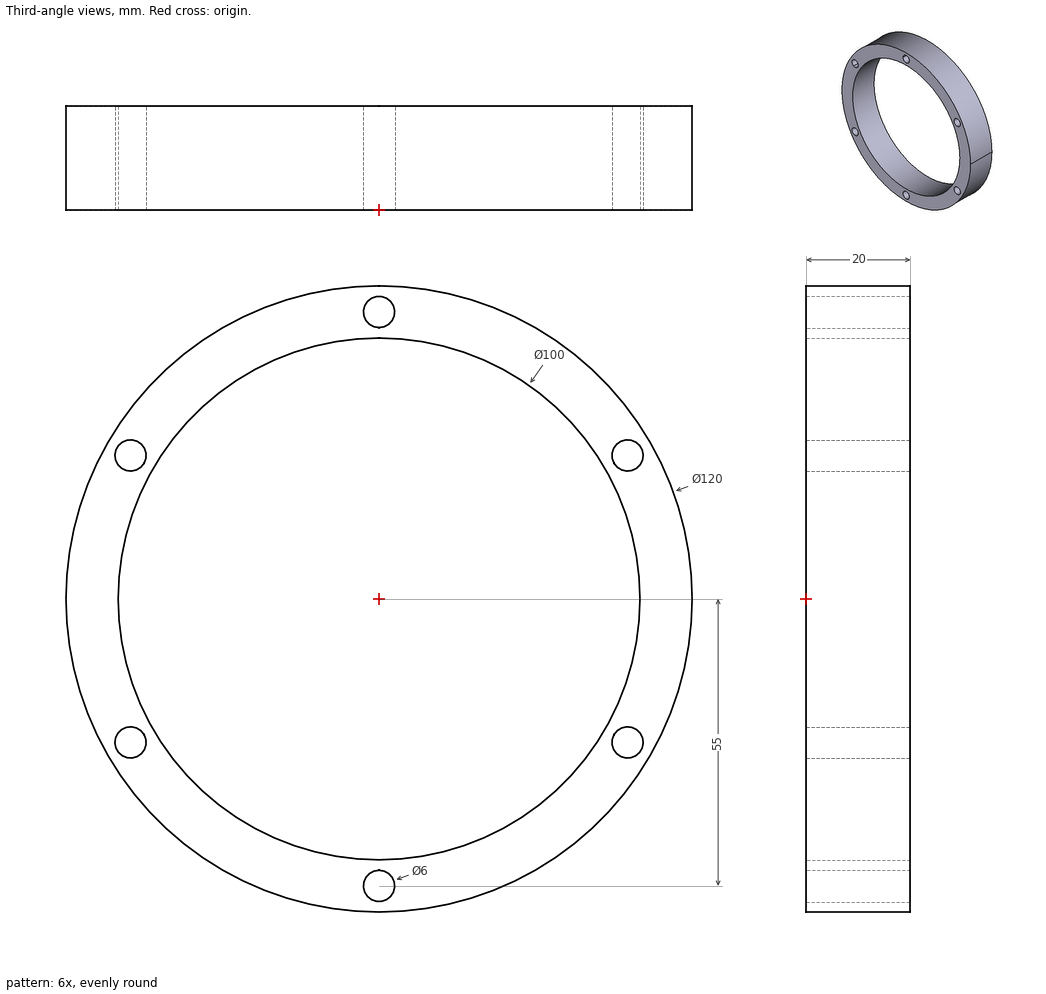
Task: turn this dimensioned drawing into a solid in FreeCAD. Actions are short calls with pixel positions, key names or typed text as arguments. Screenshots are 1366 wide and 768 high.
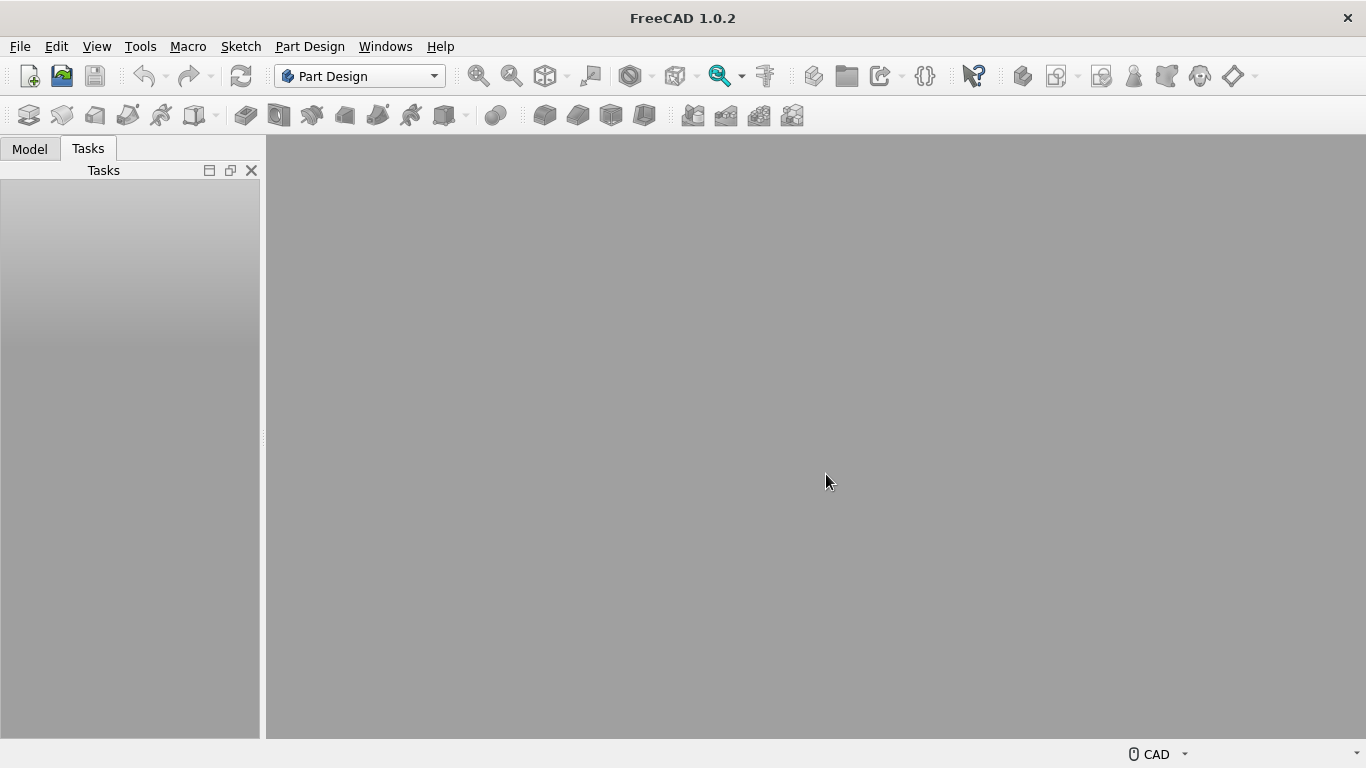
key(ctrl+n)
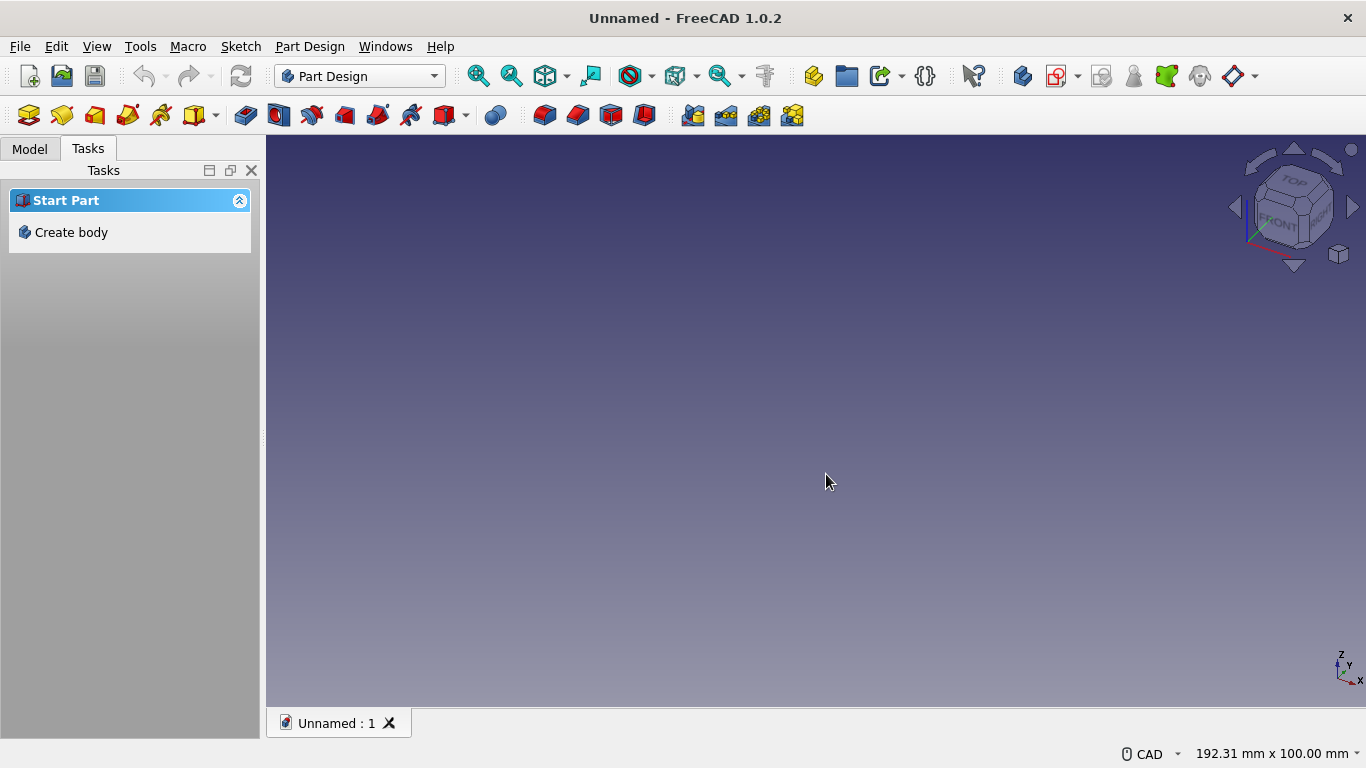
click(1056, 76)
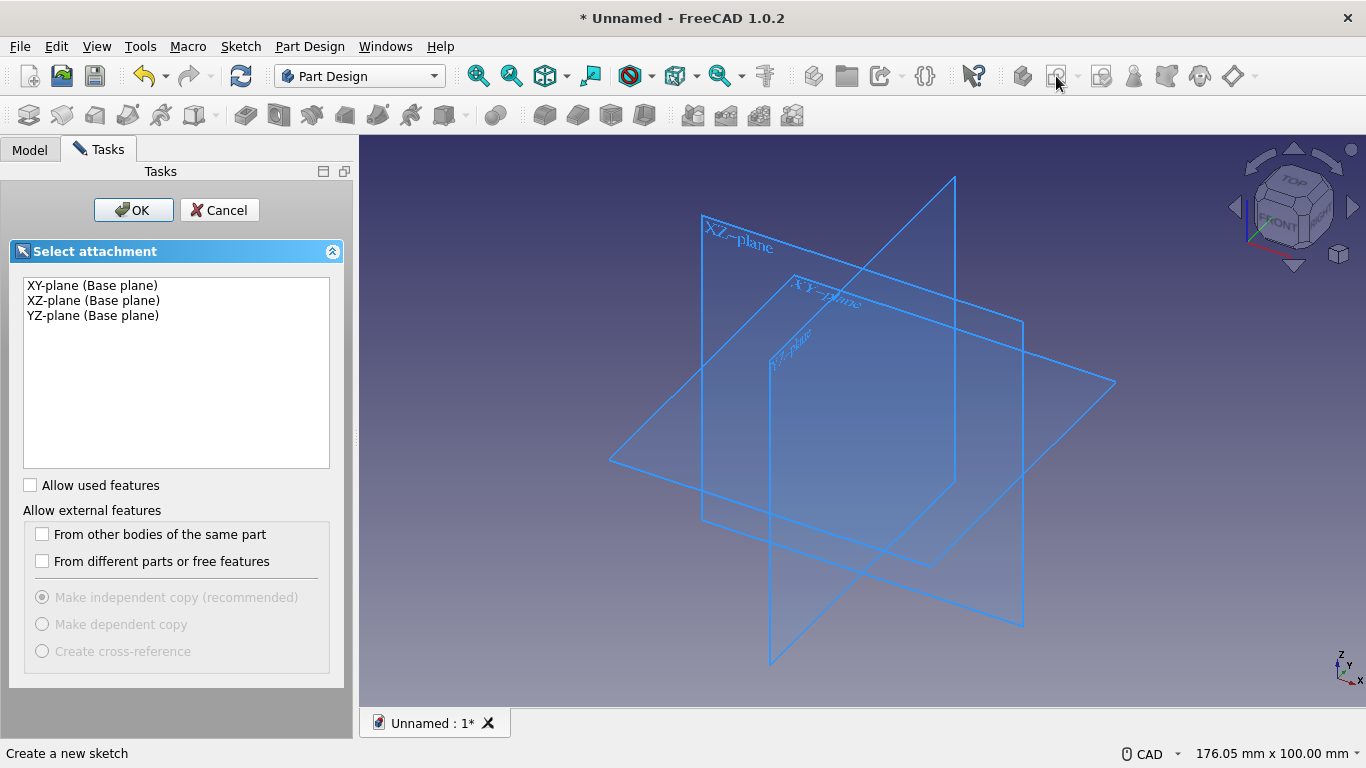
click(84, 300)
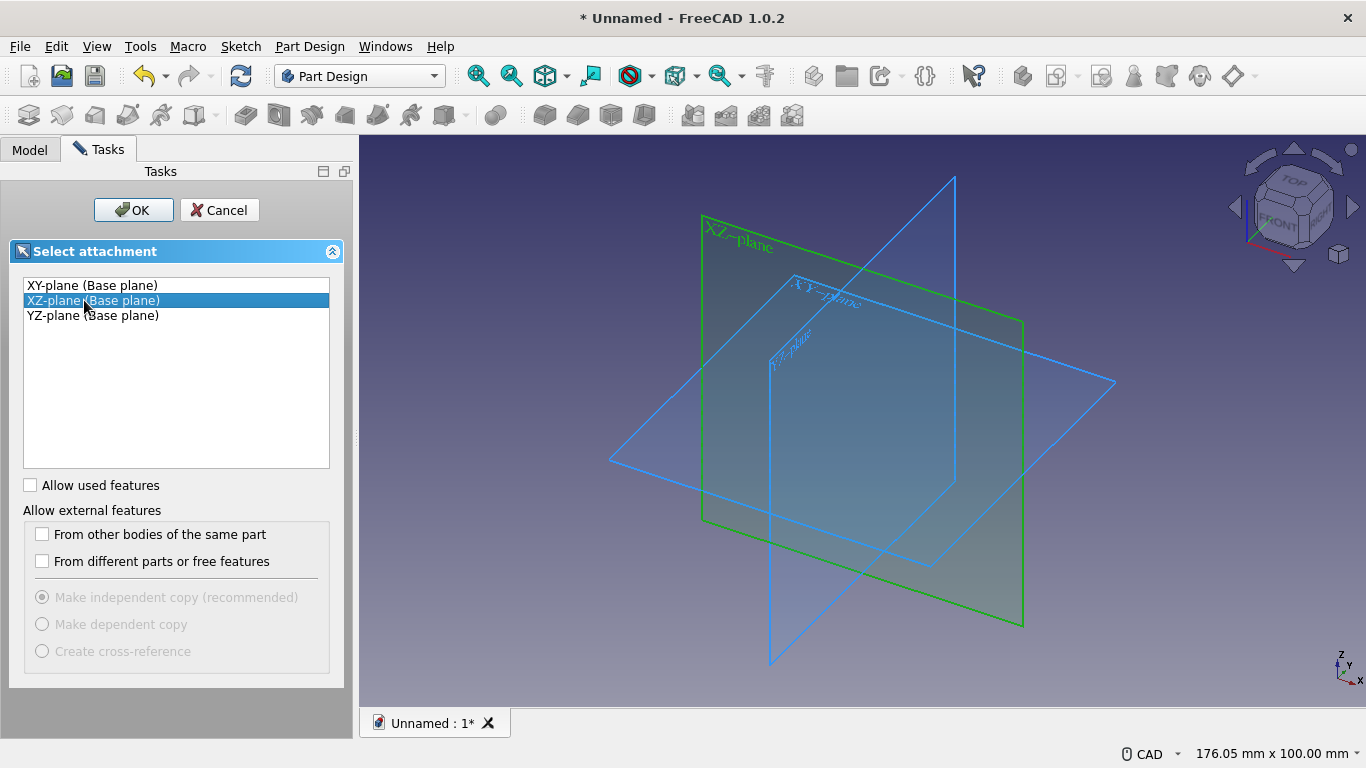
click(134, 210)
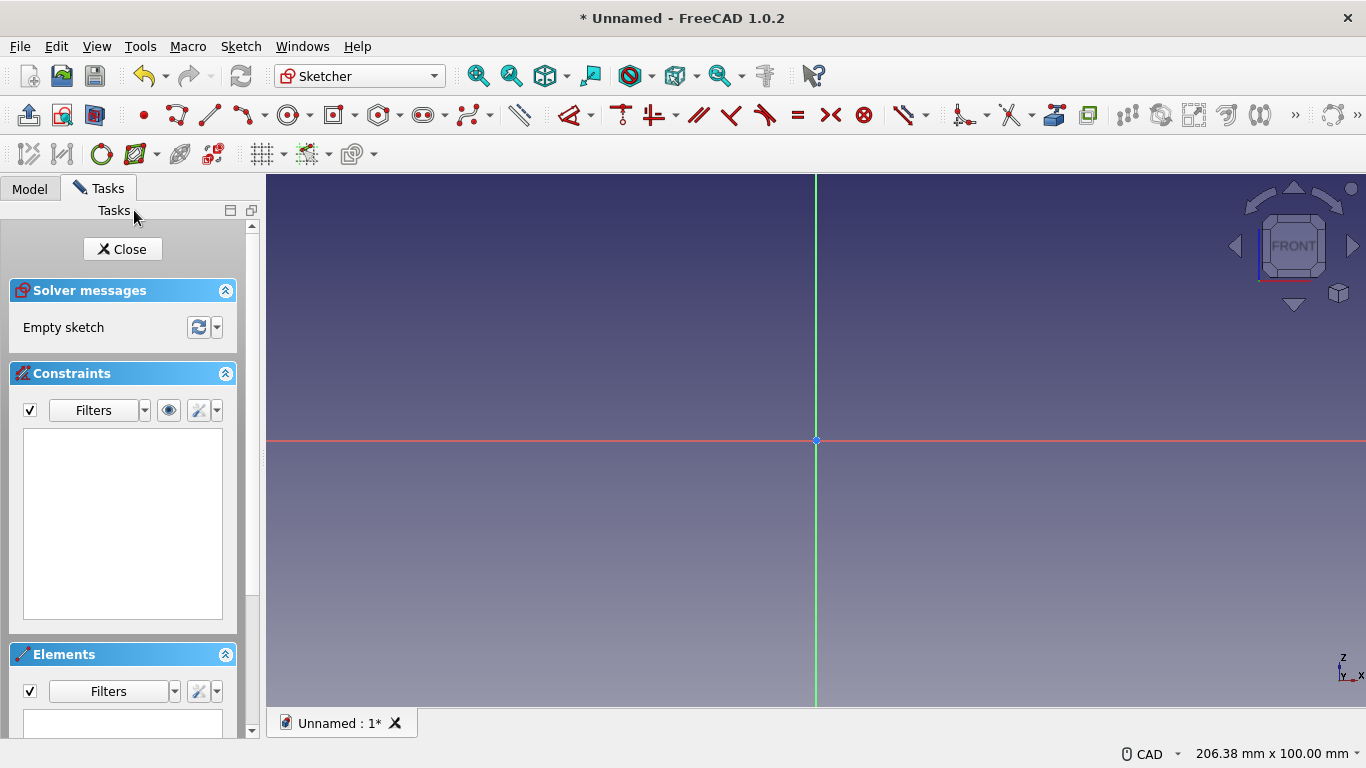
scroll(664, 440, down, 3)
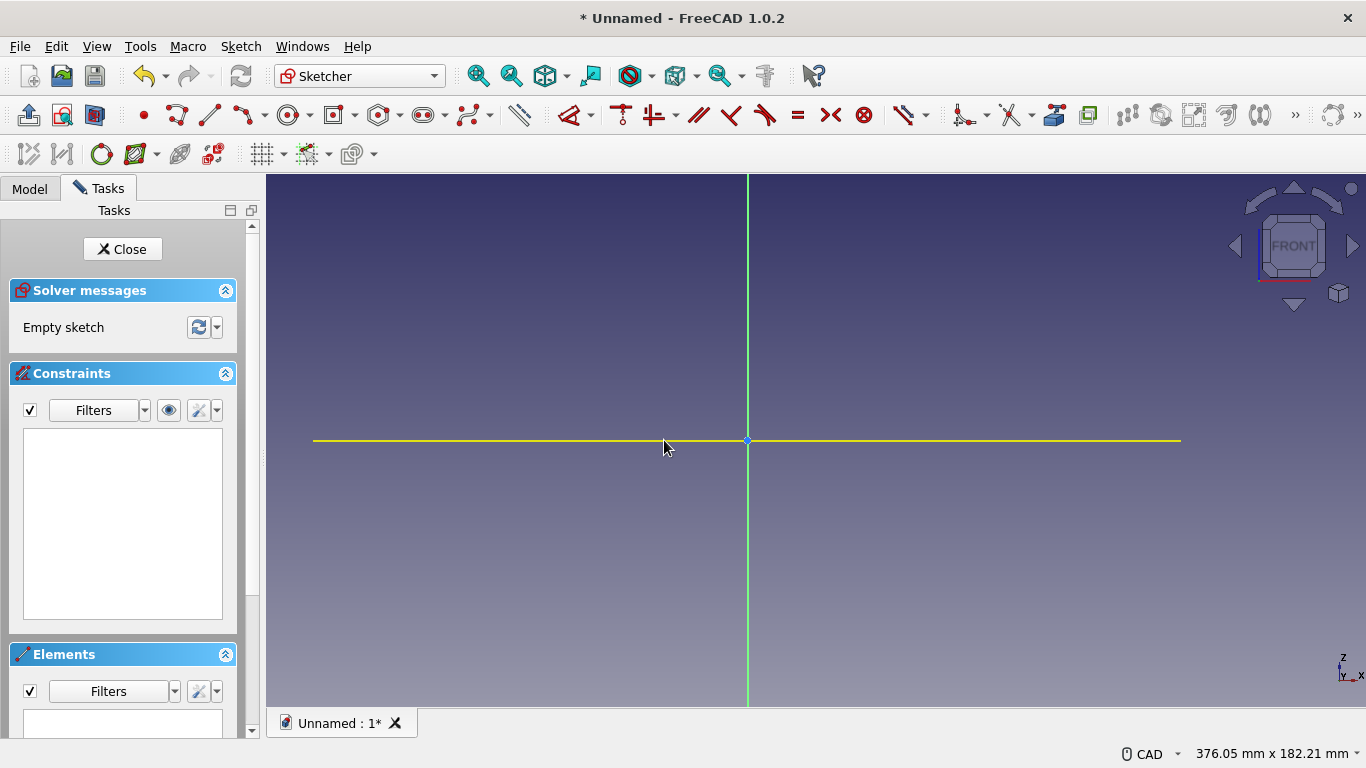
click(288, 116)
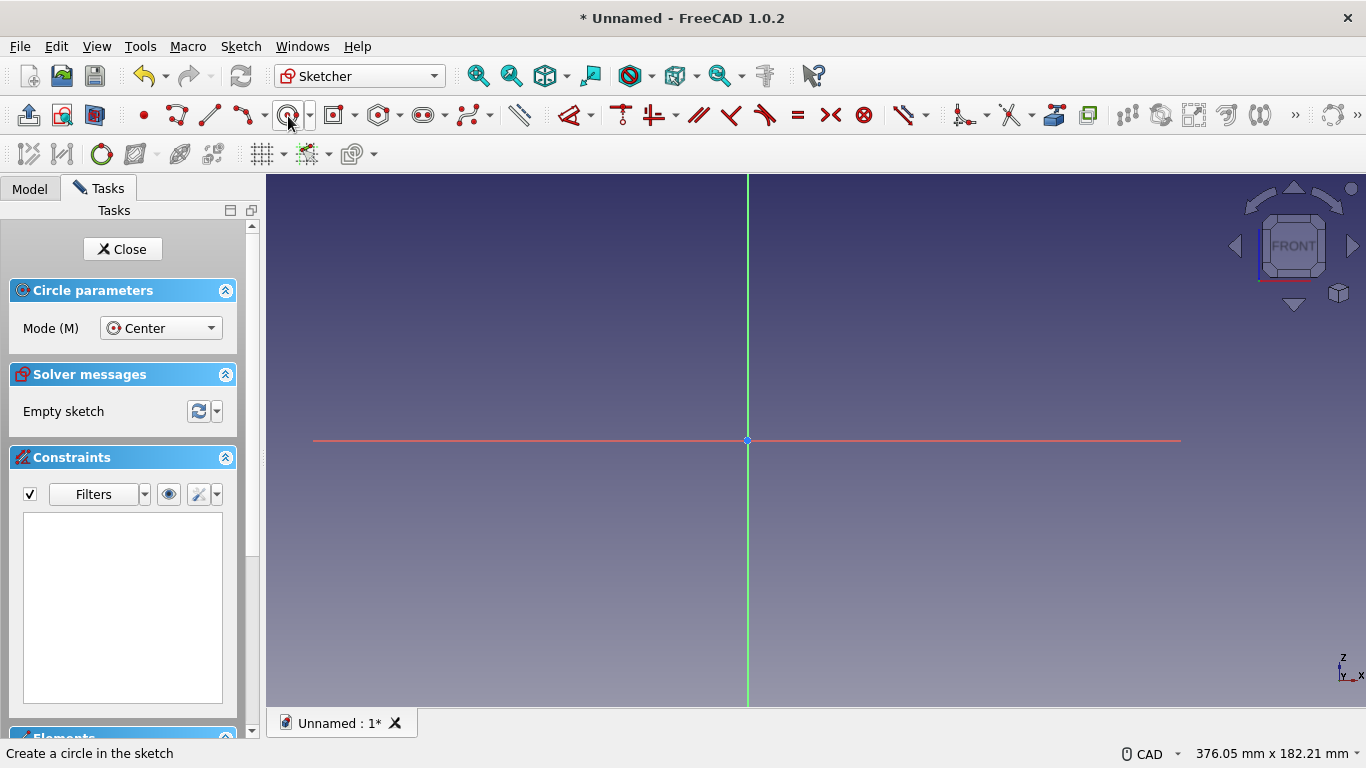
click(748, 440)
move(872, 316)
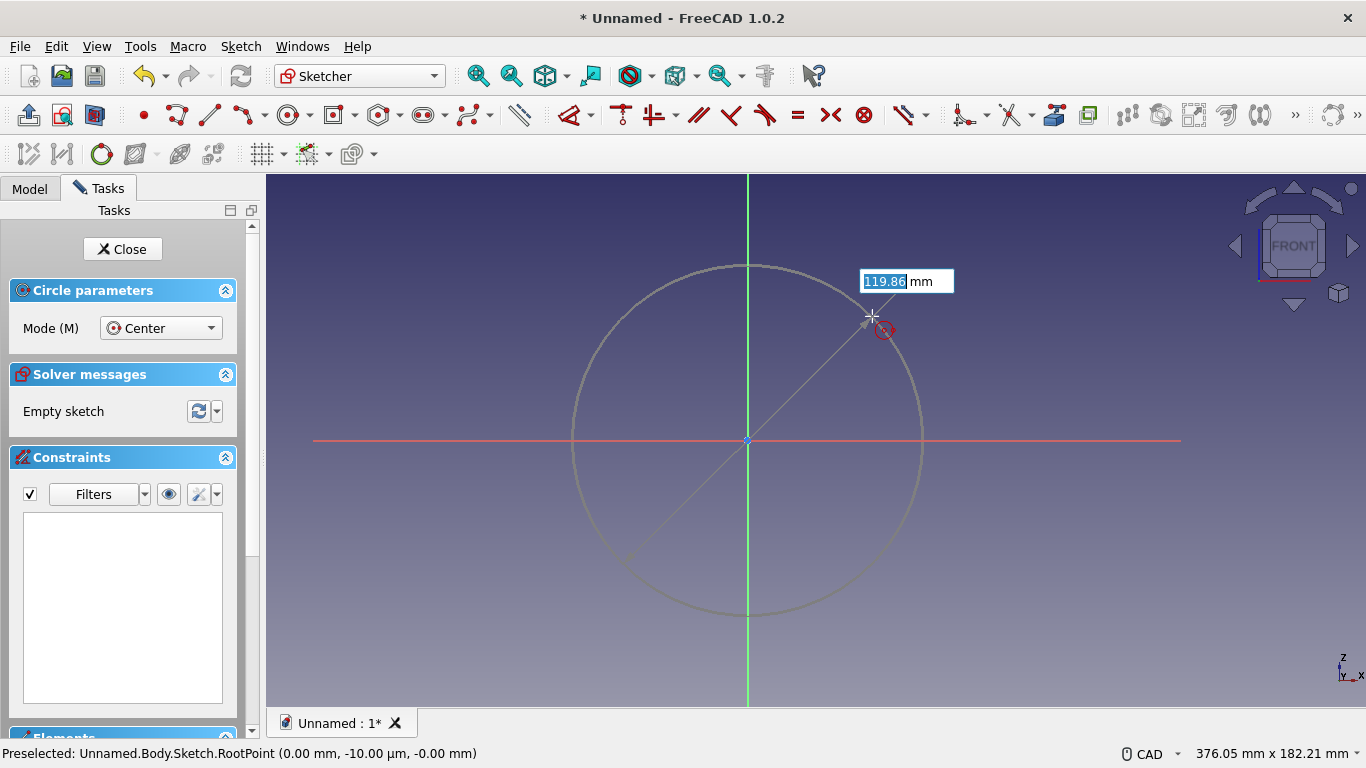
text(120)
key(Return)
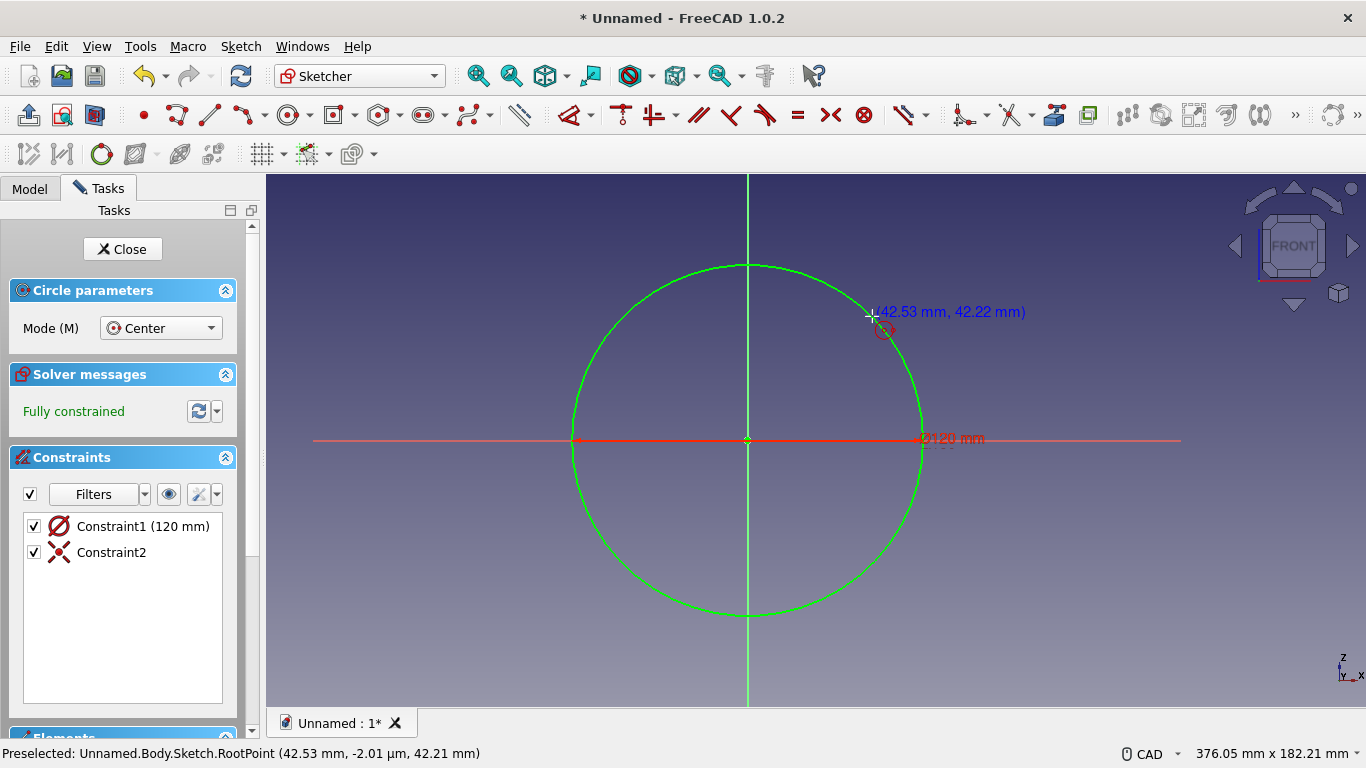
click(748, 440)
move(851, 337)